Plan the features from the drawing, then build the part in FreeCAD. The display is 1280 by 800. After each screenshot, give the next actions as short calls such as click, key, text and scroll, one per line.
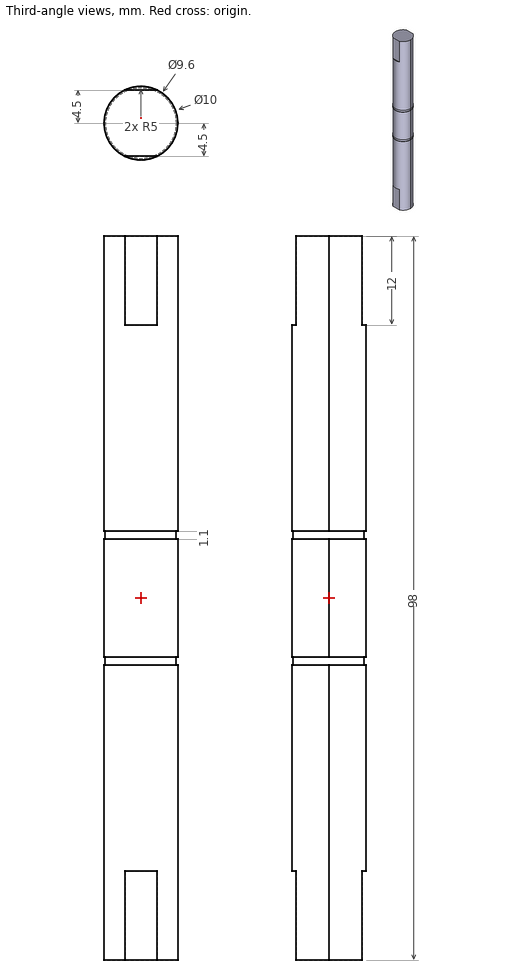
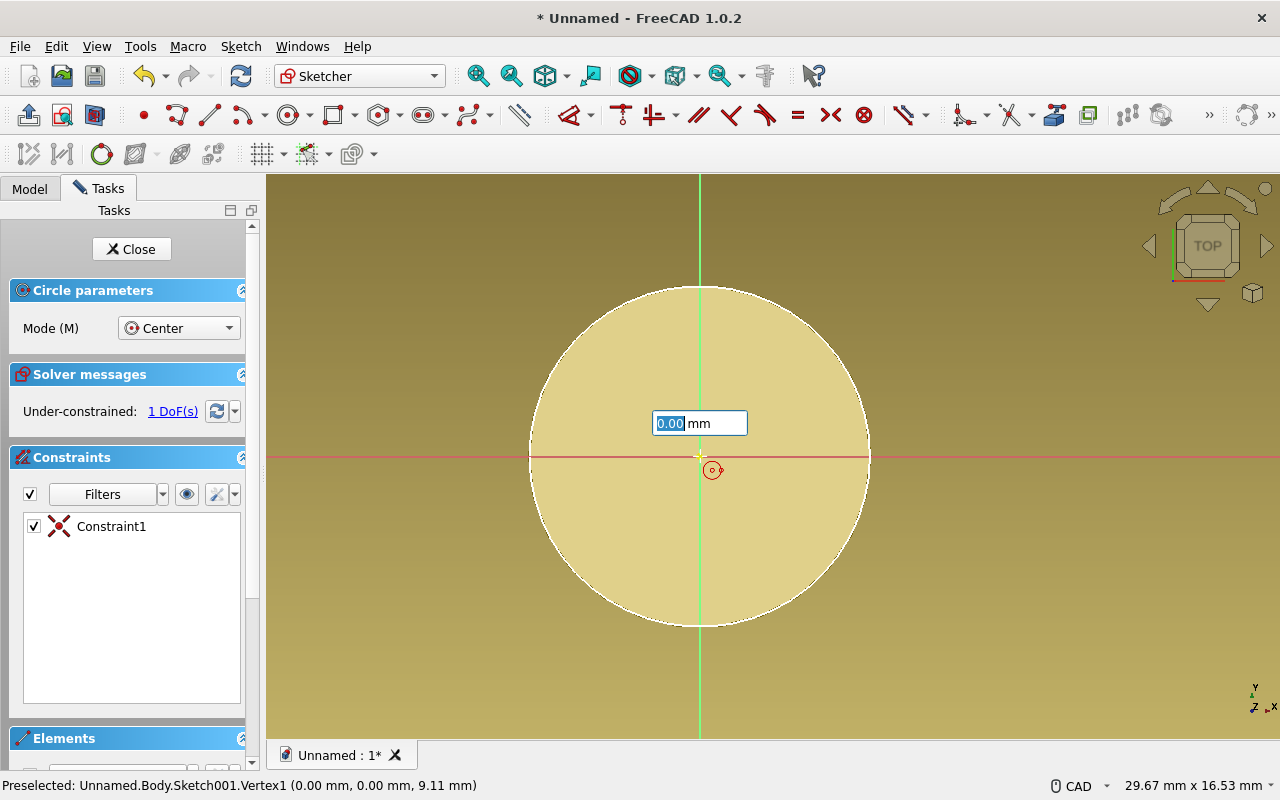
scroll(816, 340, up, 5)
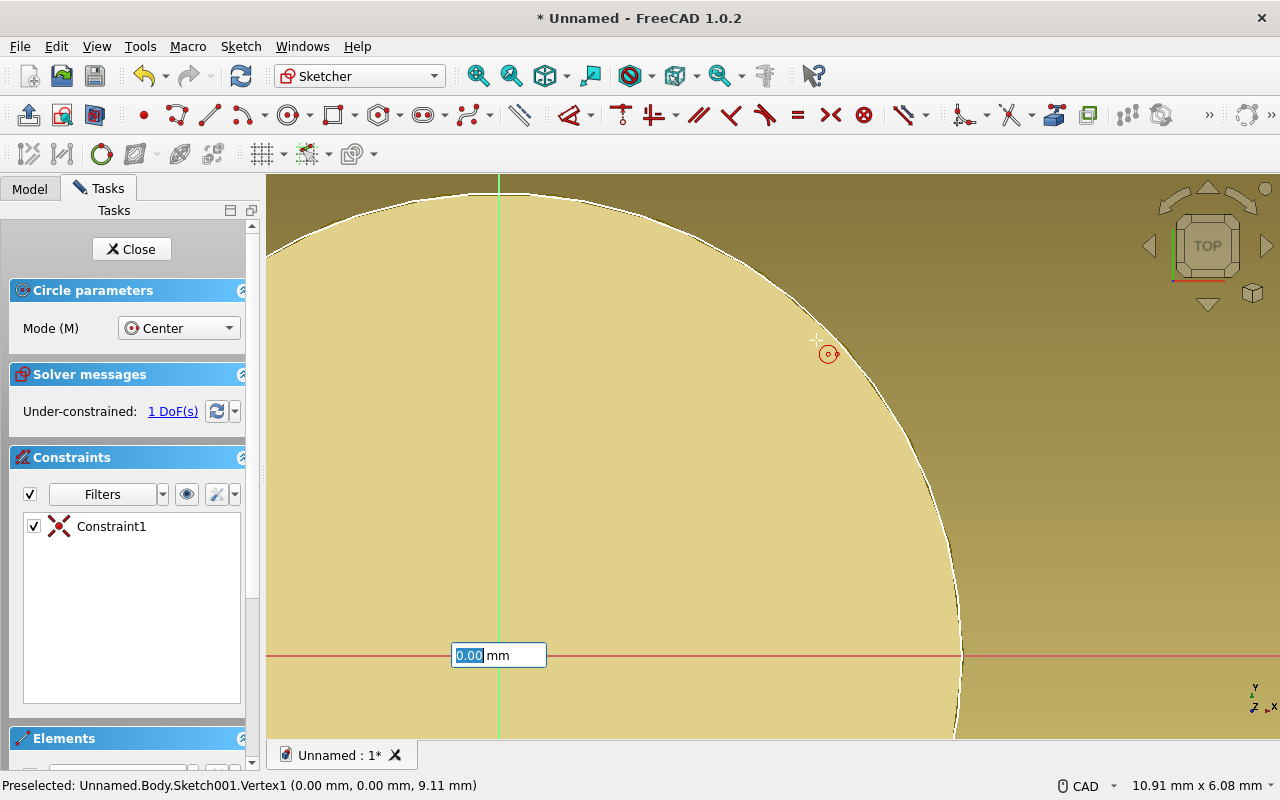
click(814, 341)
key(Escape)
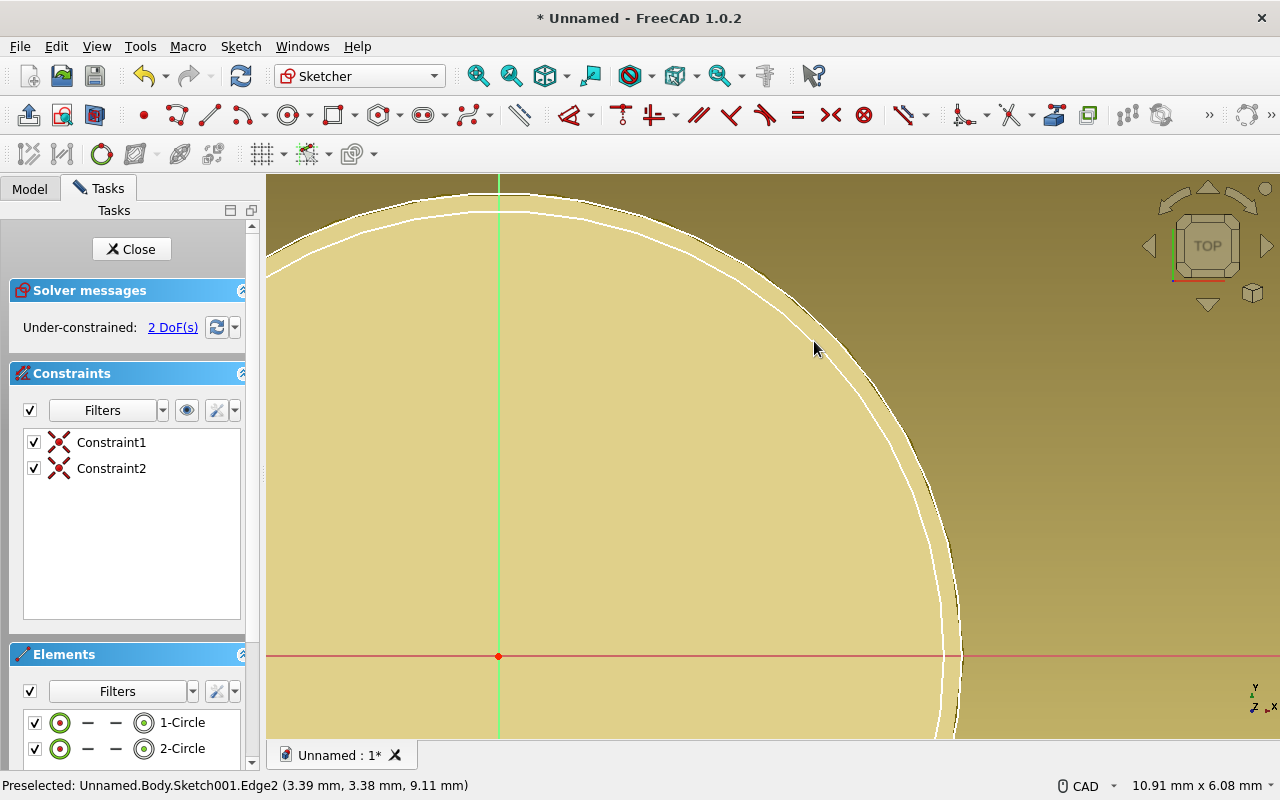
click(568, 116)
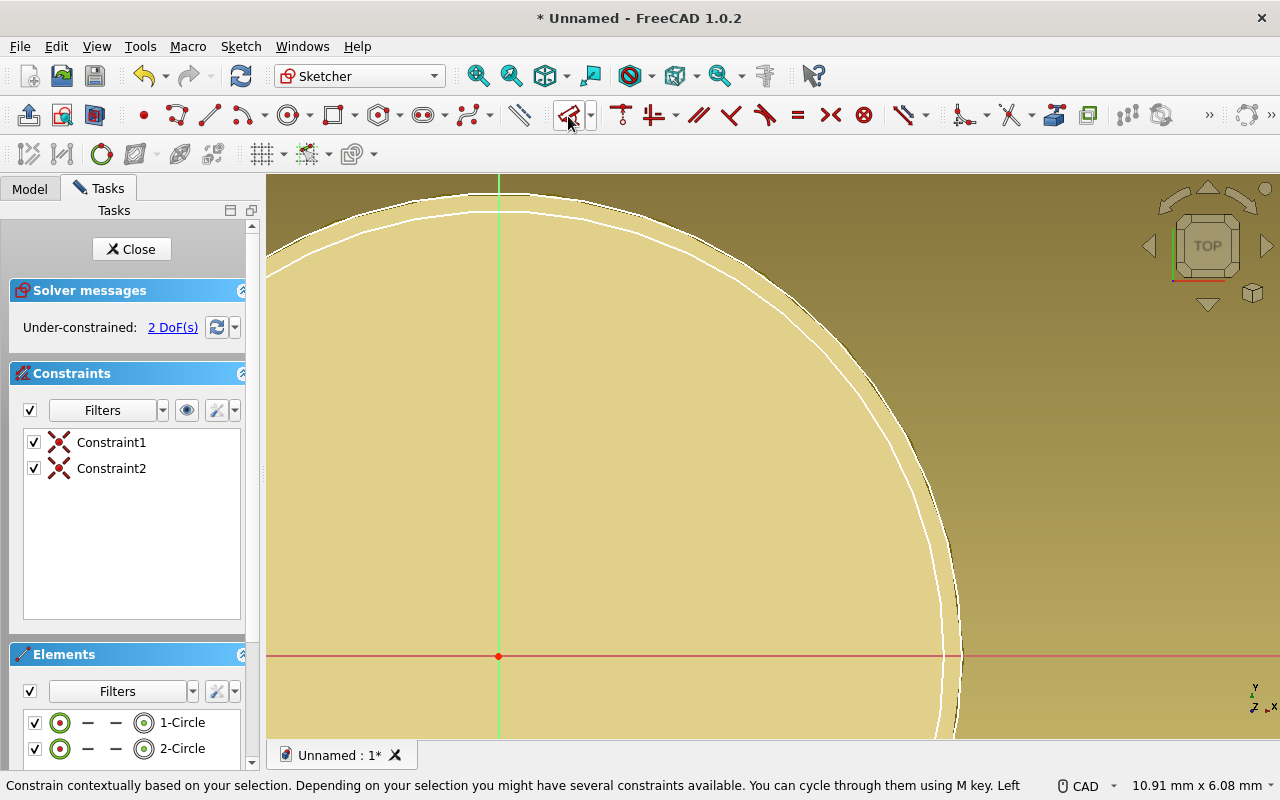
click(825, 328)
click(848, 305)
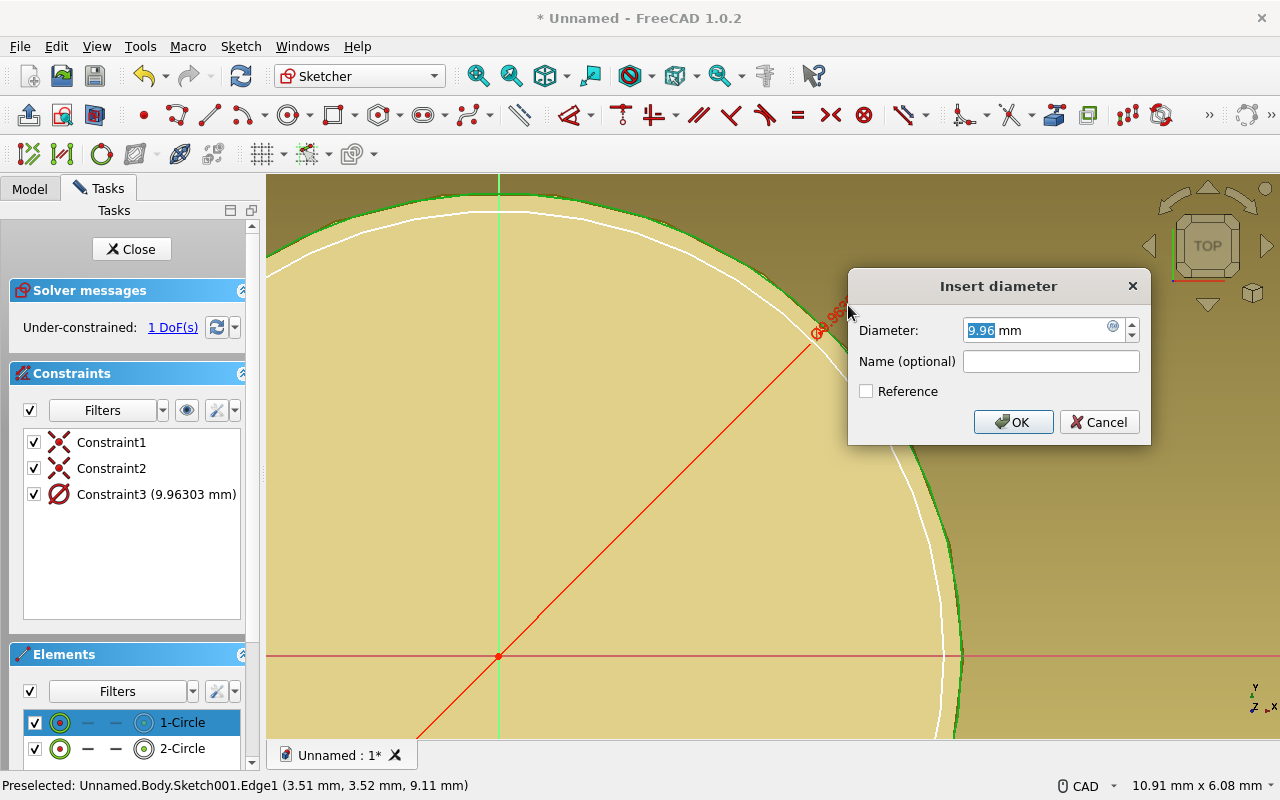
text(10)
key(Return)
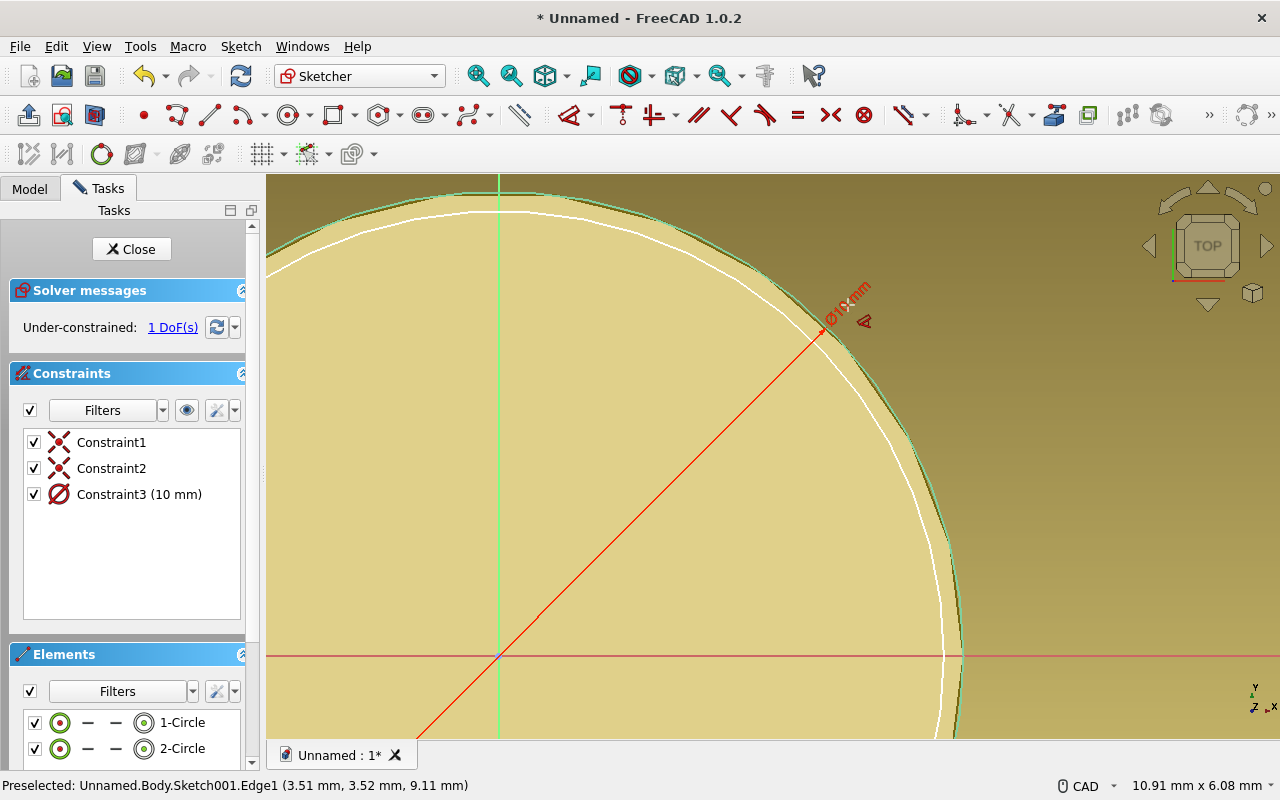
click(813, 341)
click(978, 515)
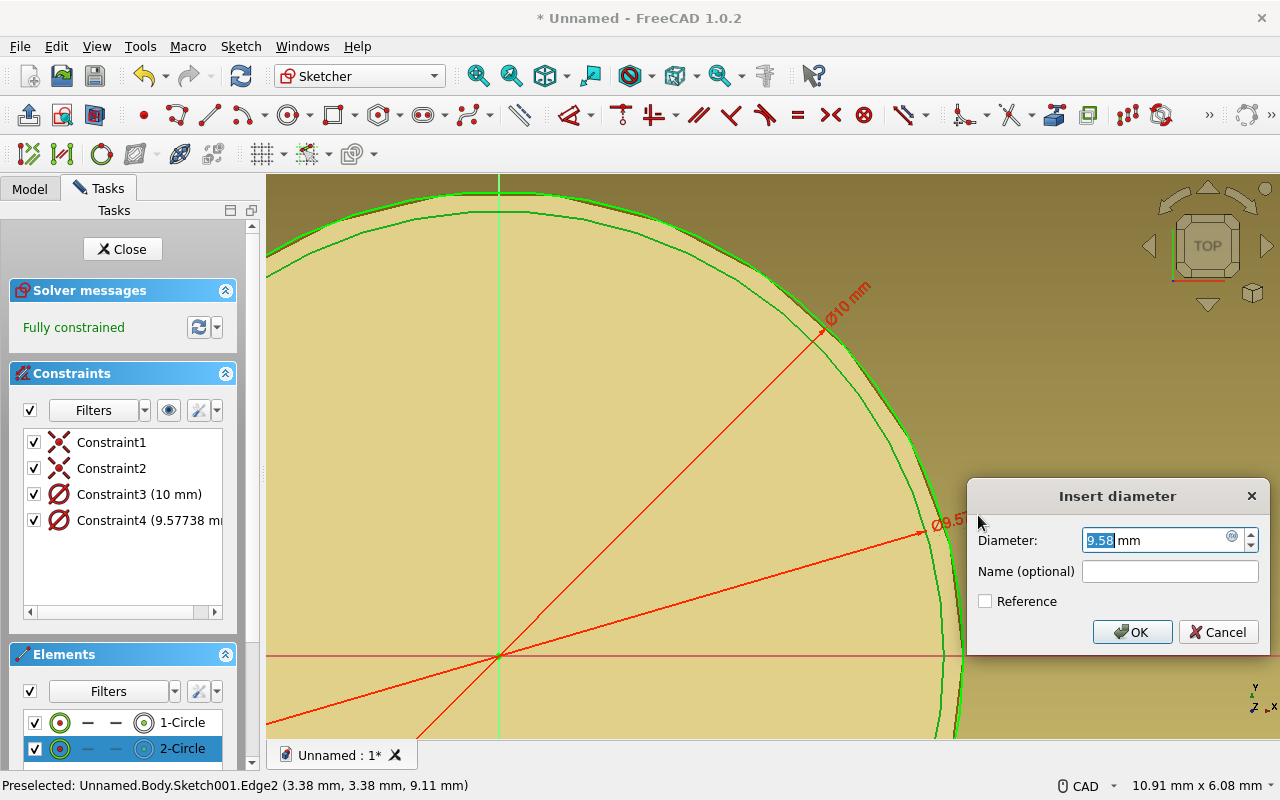
text(9.6)
key(Return)
key(Escape)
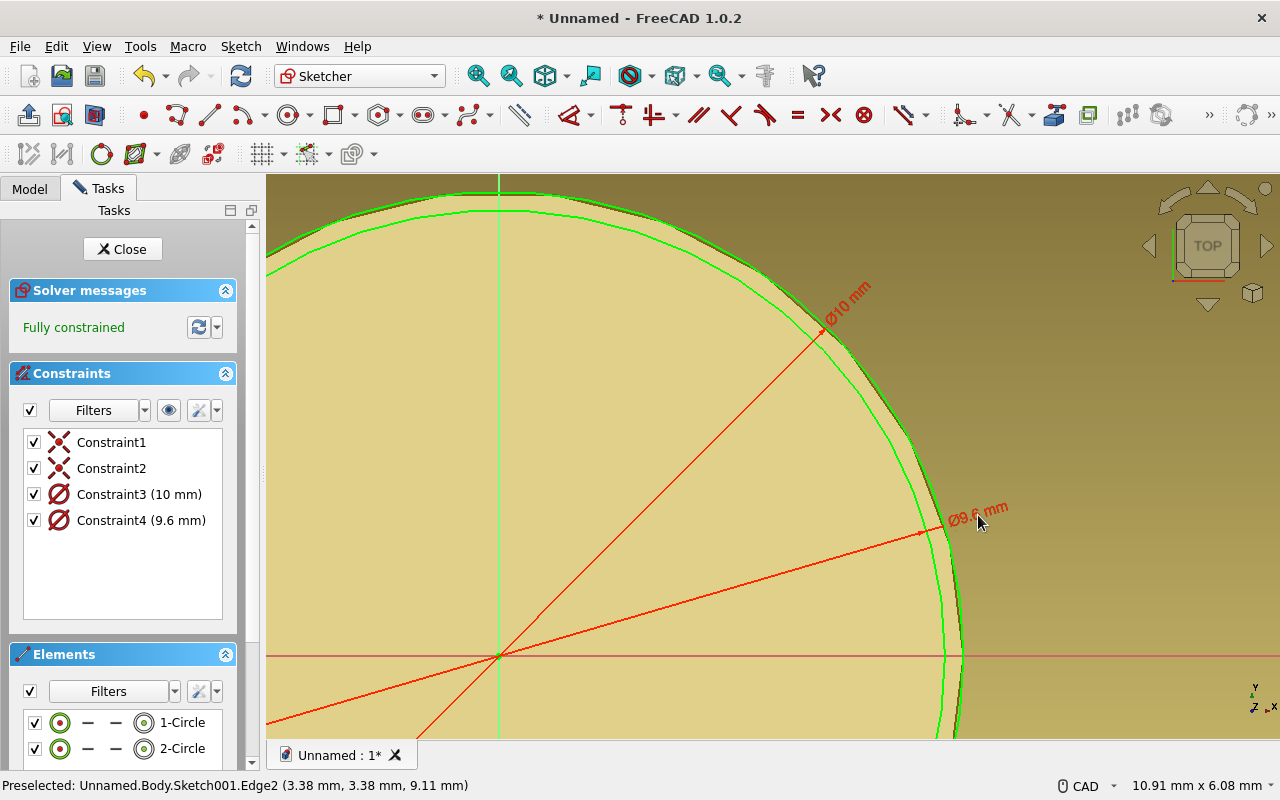
click(123, 249)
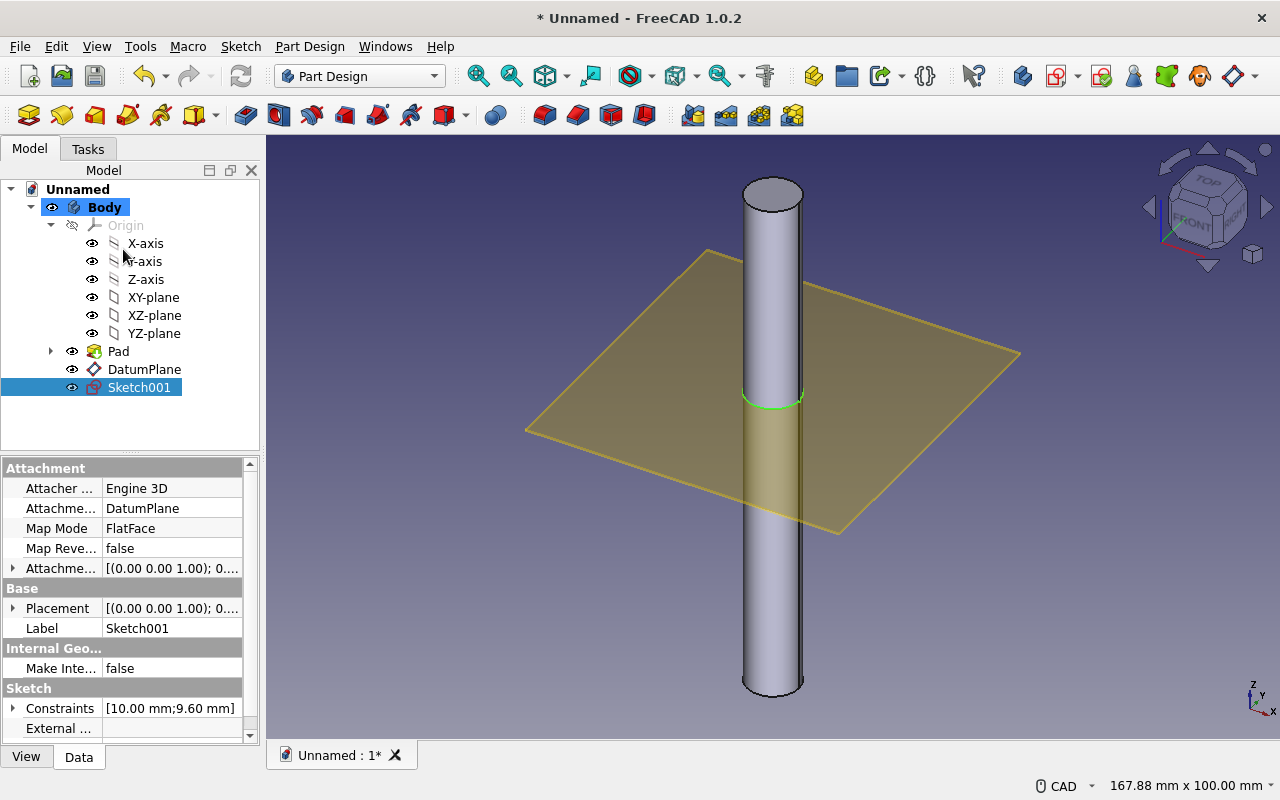
click(246, 116)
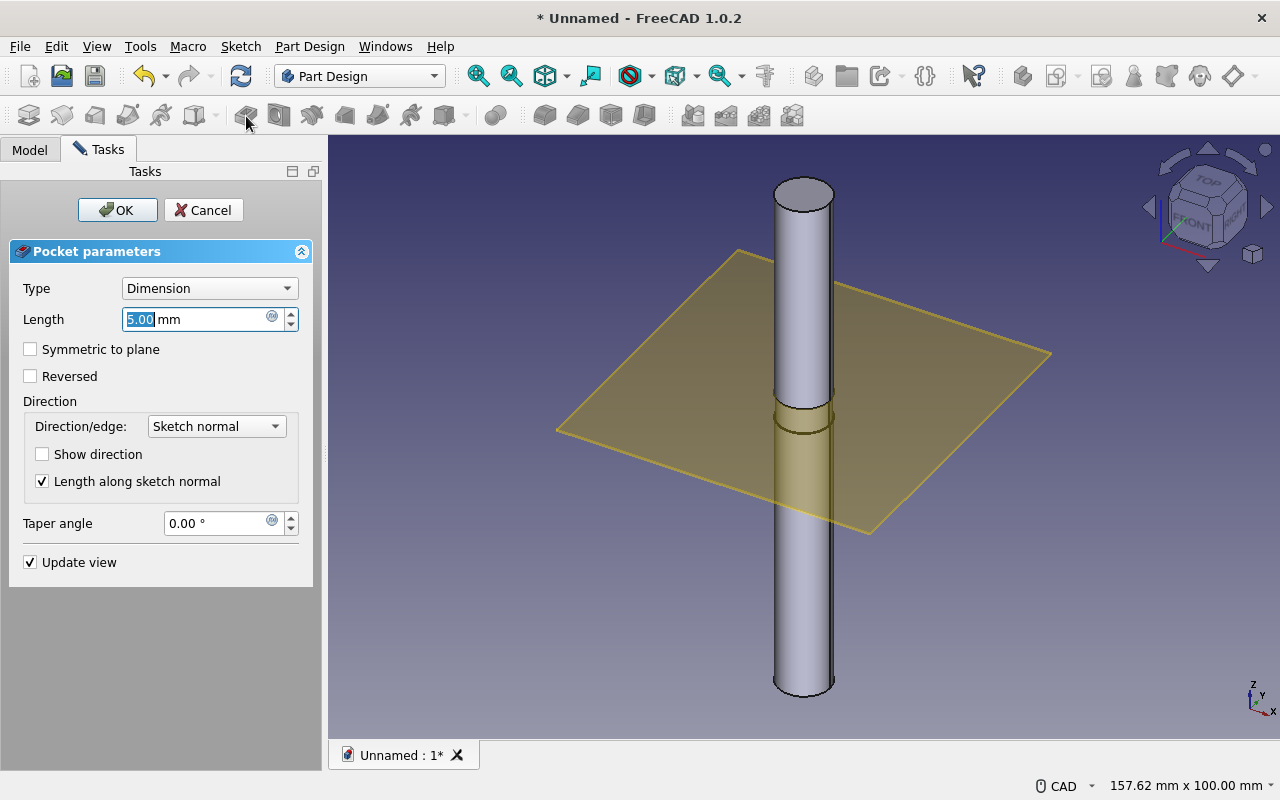
text(1.1)
key(Tab)